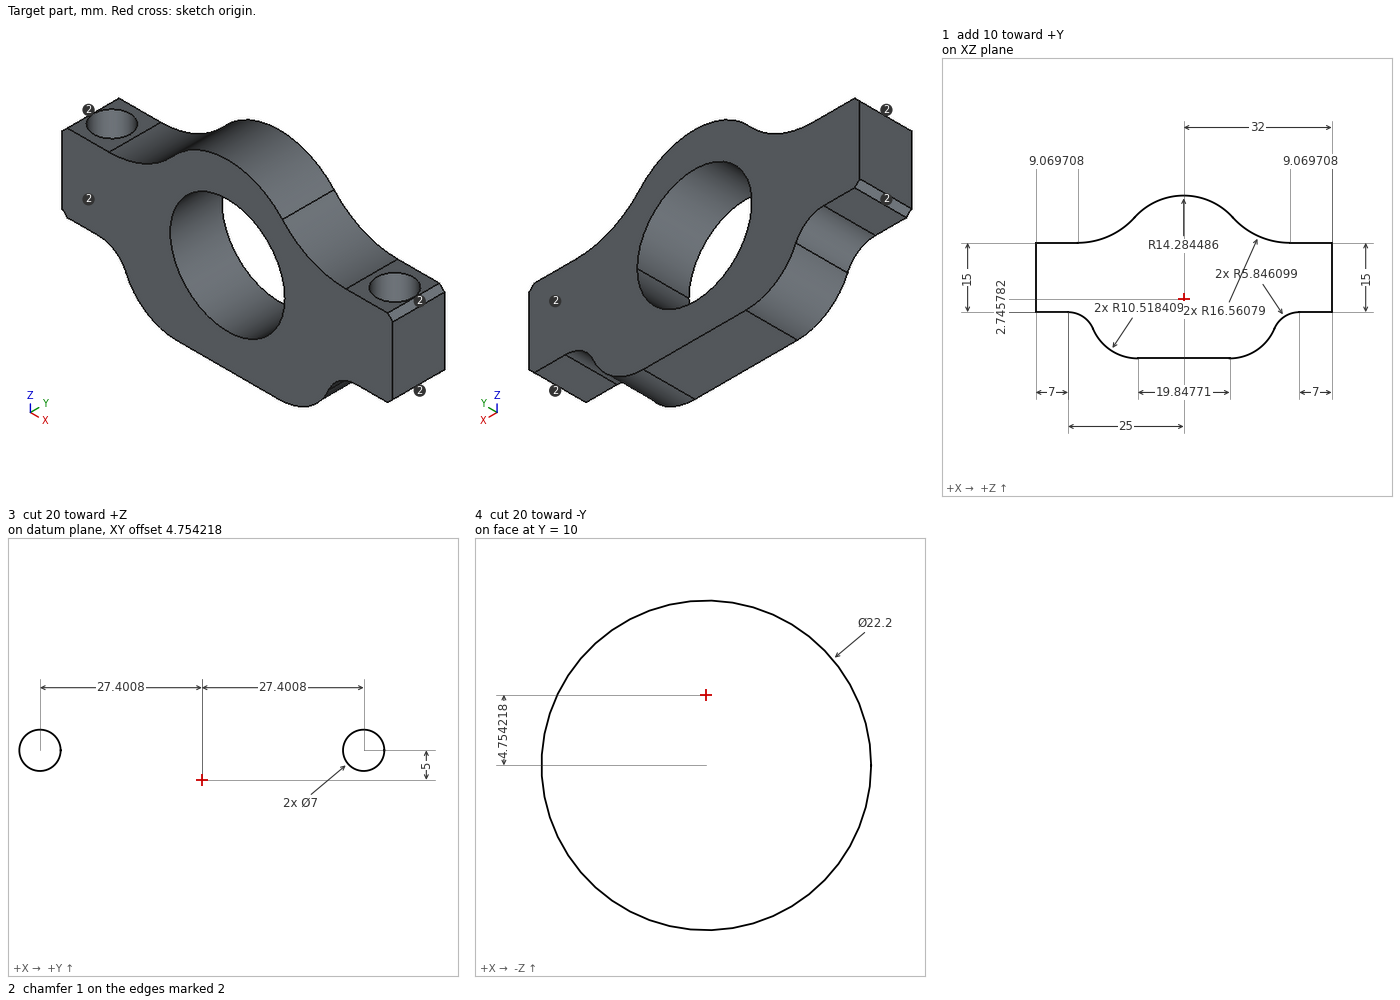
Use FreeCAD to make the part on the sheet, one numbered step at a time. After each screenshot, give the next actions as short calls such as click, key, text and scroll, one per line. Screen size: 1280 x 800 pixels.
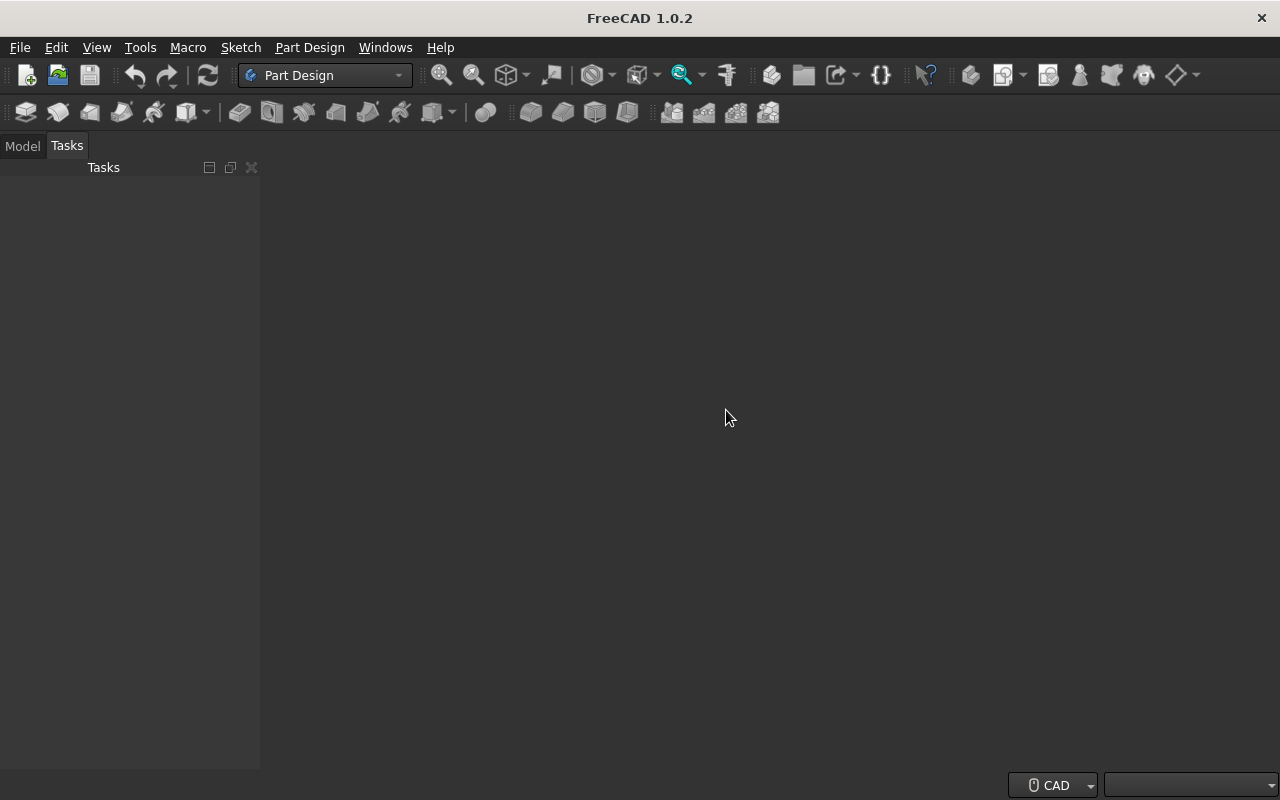
click(26, 76)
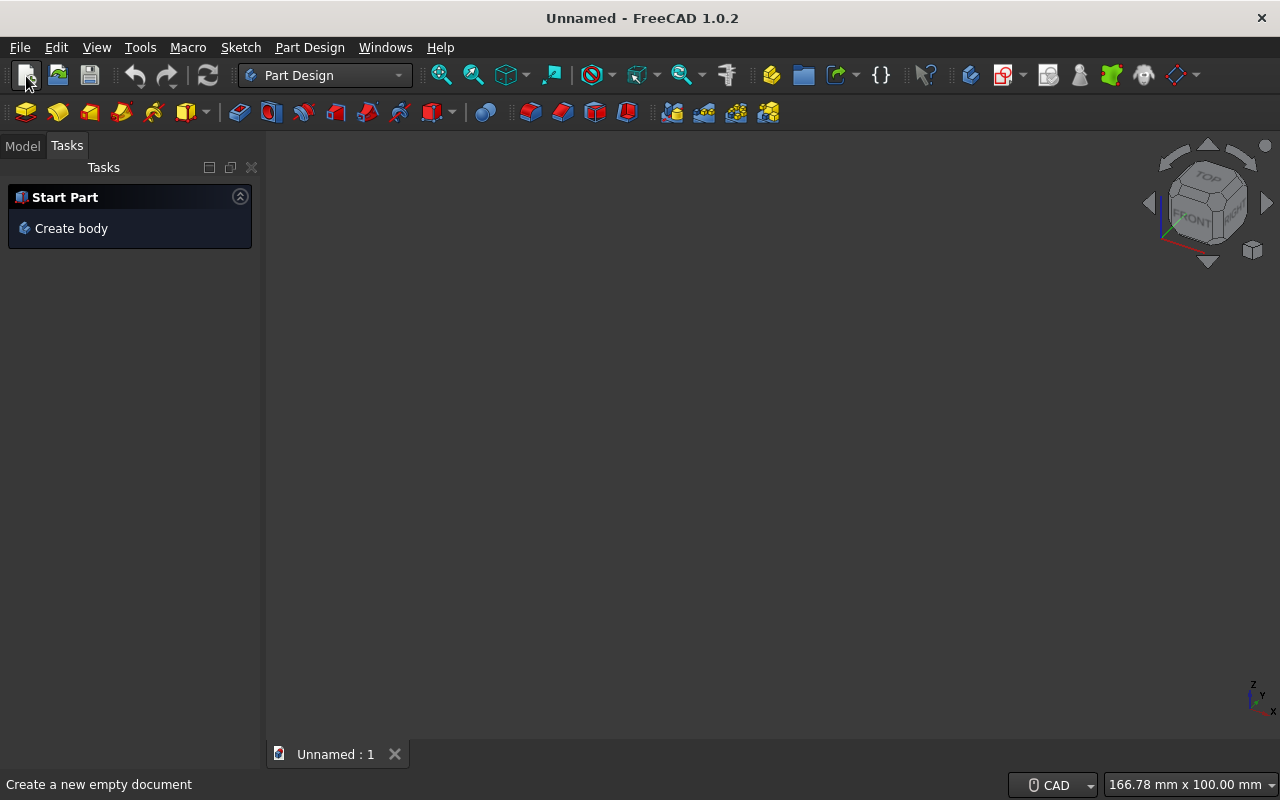
click(1004, 76)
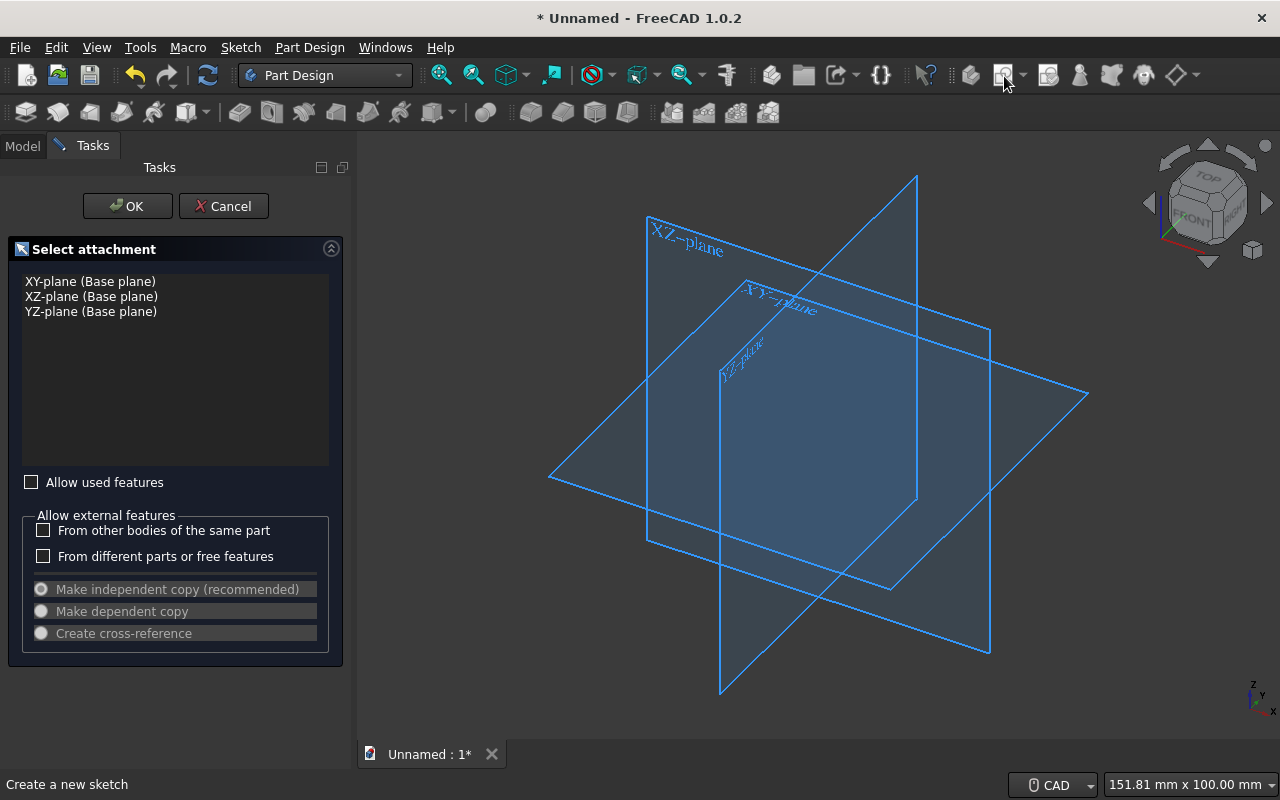
click(82, 296)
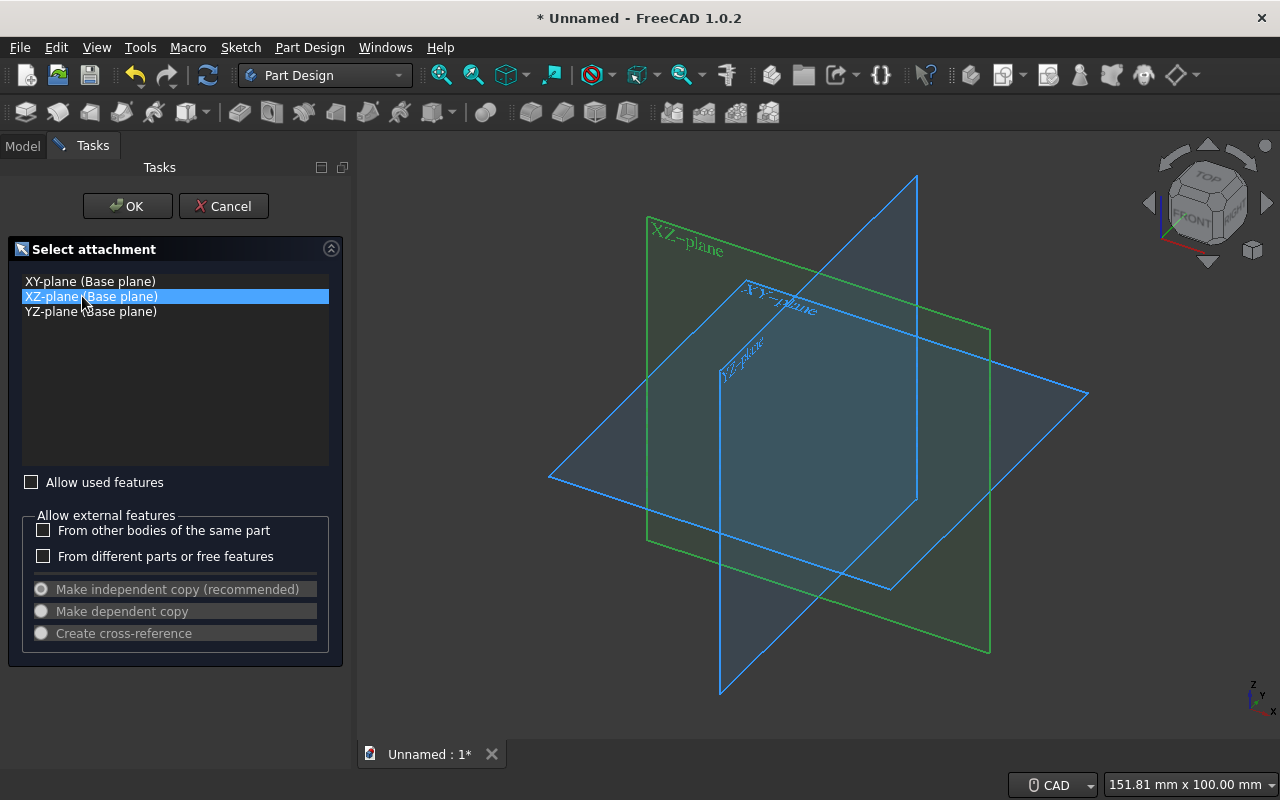
click(128, 206)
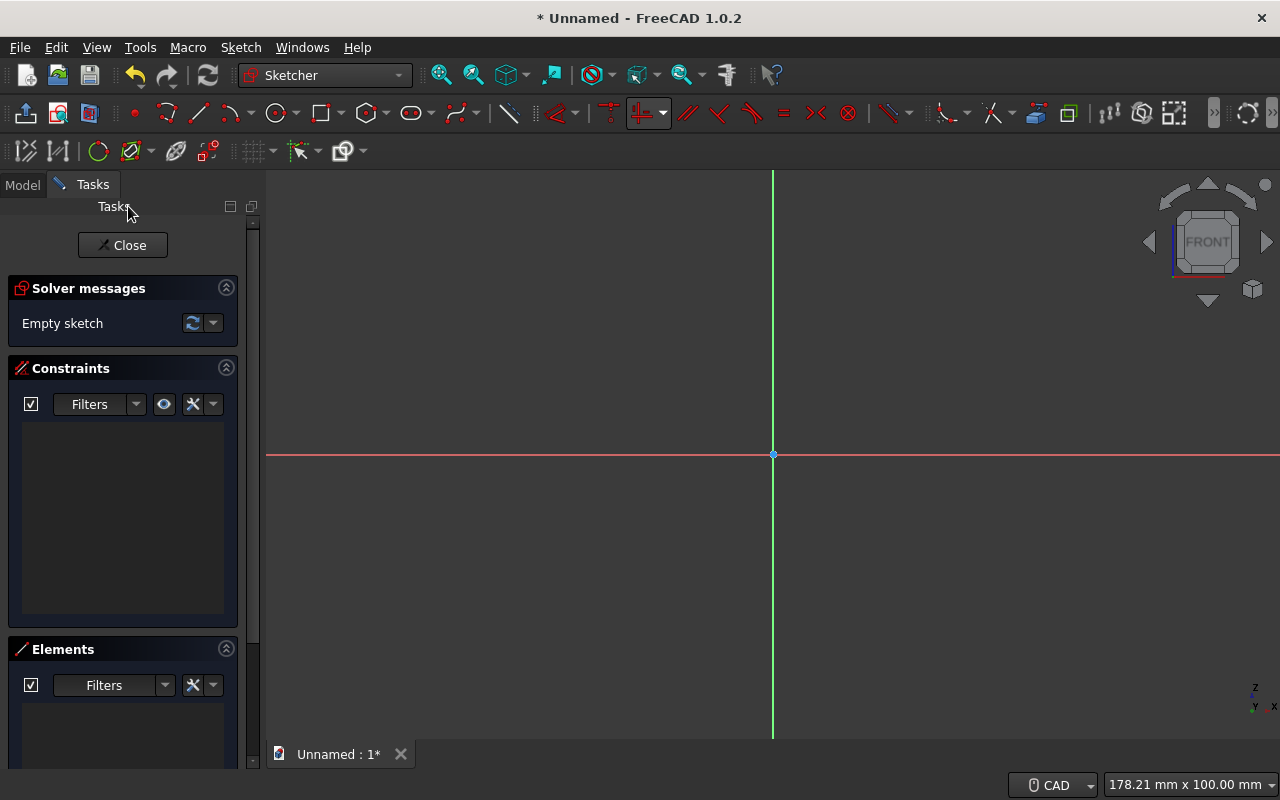
scroll(912, 371, up, 2)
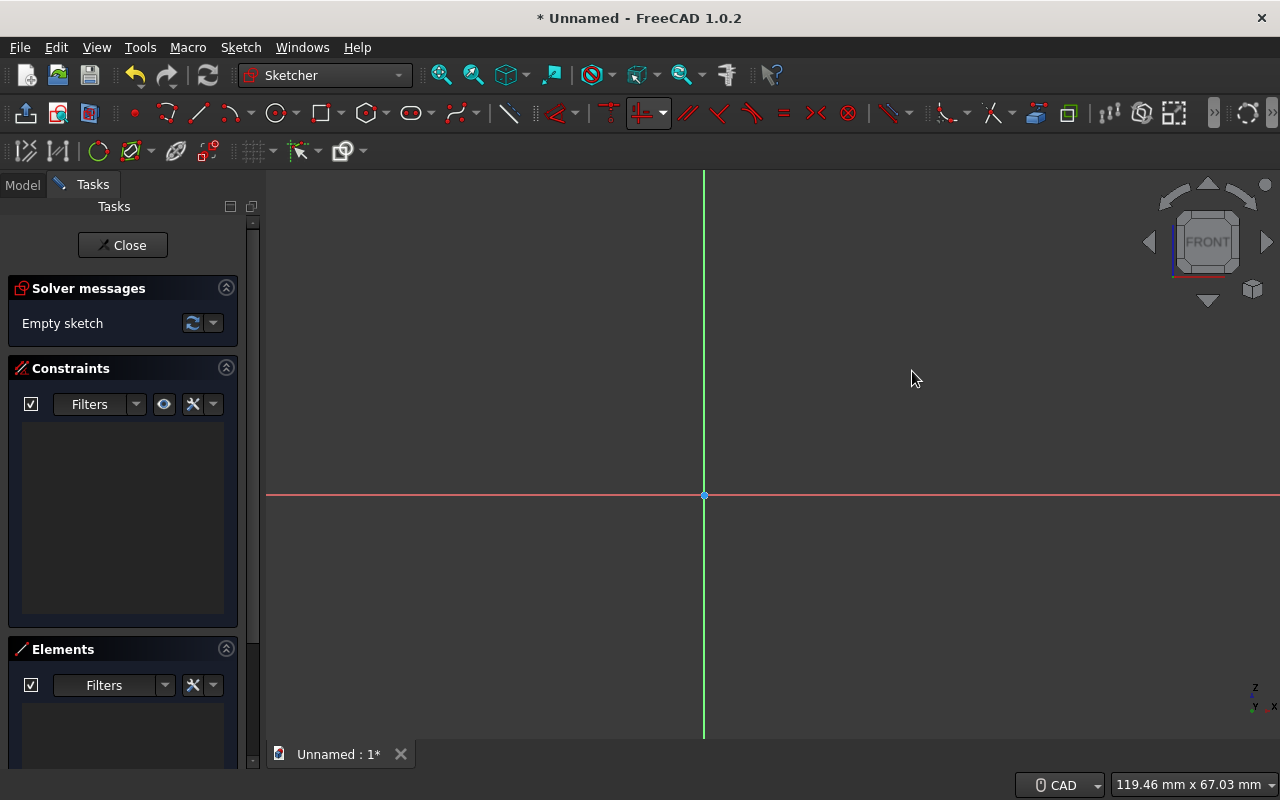
click(200, 114)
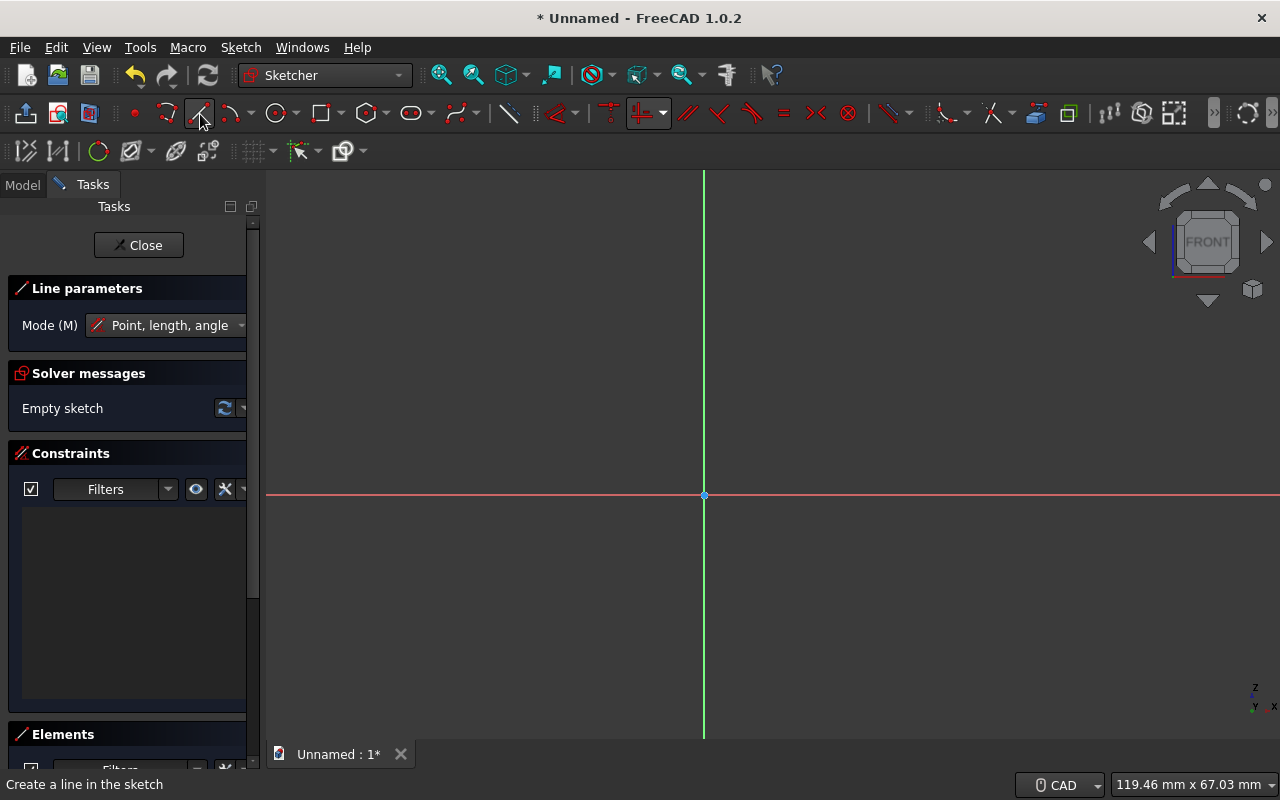
click(789, 604)
click(620, 604)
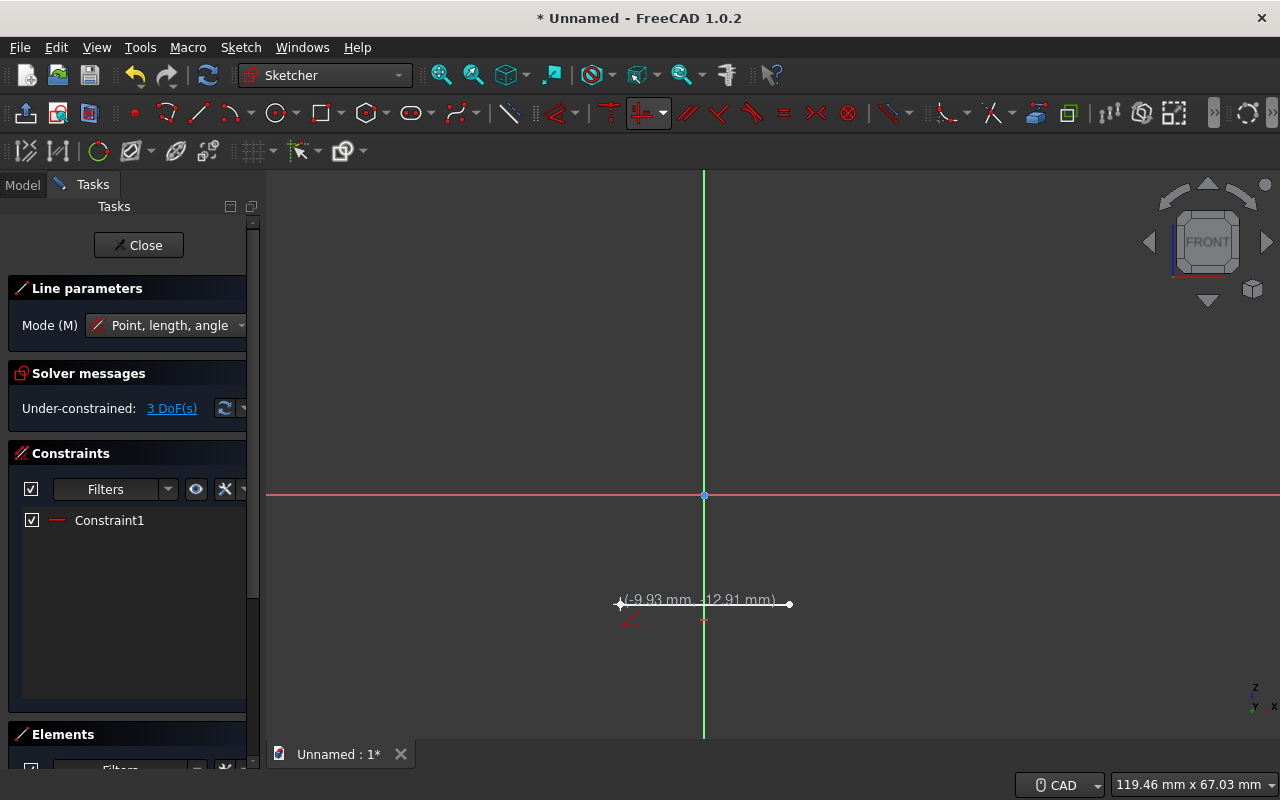
click(168, 114)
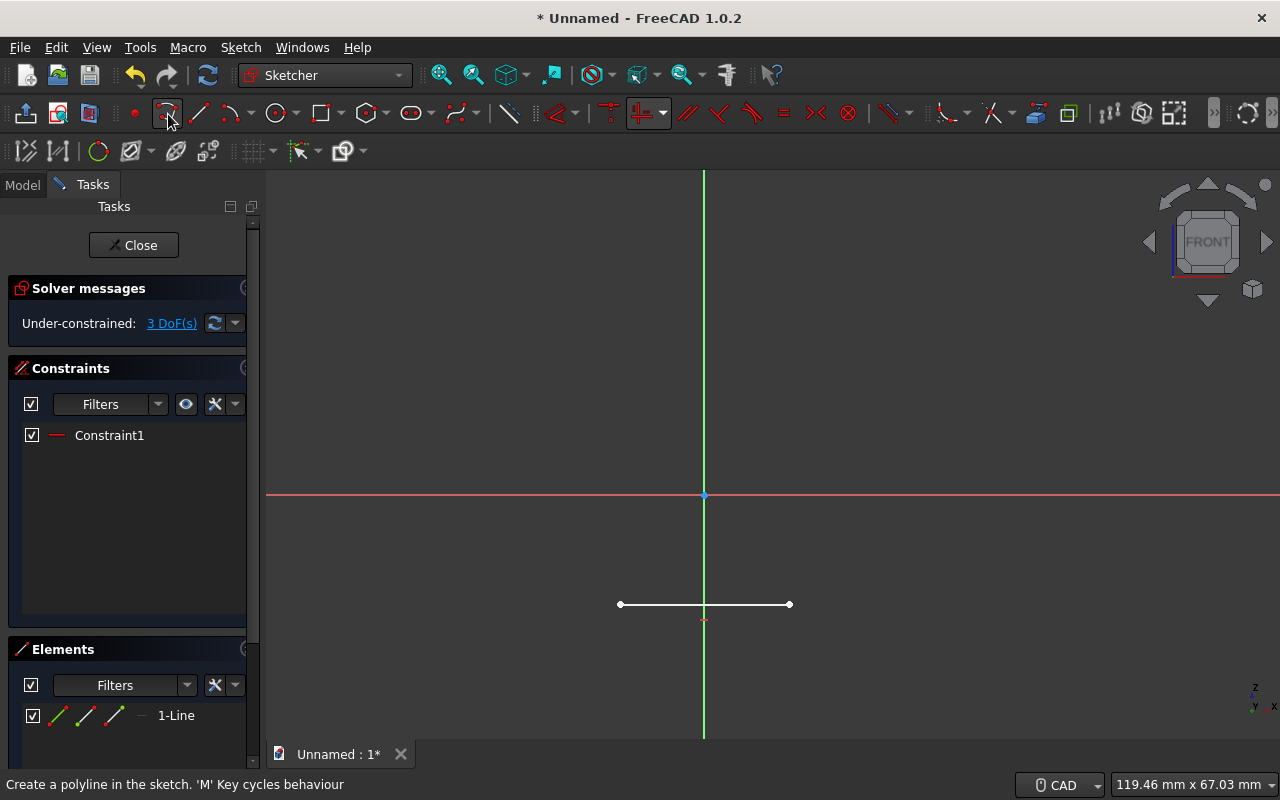
click(492, 519)
click(433, 519)
click(433, 391)
click(510, 391)
right_click(510, 391)